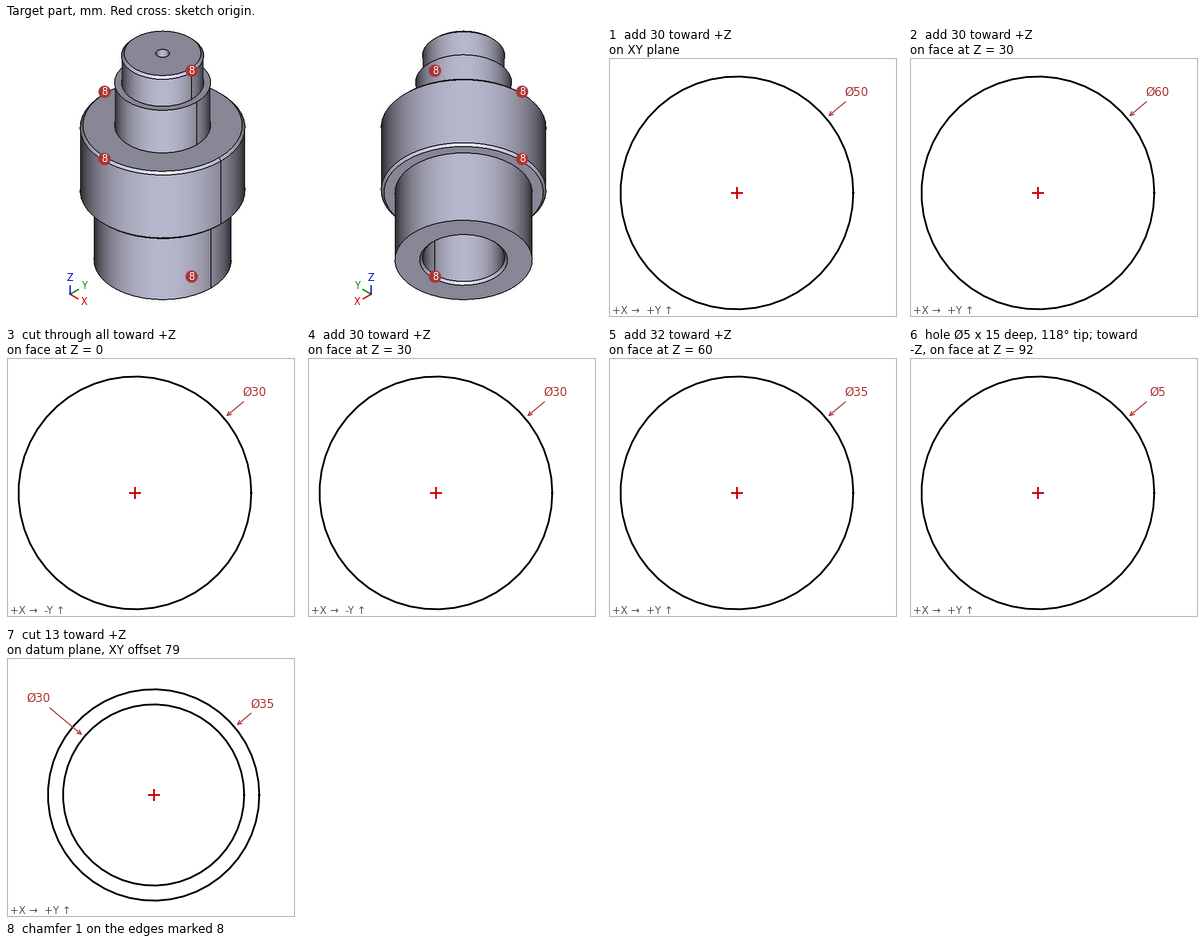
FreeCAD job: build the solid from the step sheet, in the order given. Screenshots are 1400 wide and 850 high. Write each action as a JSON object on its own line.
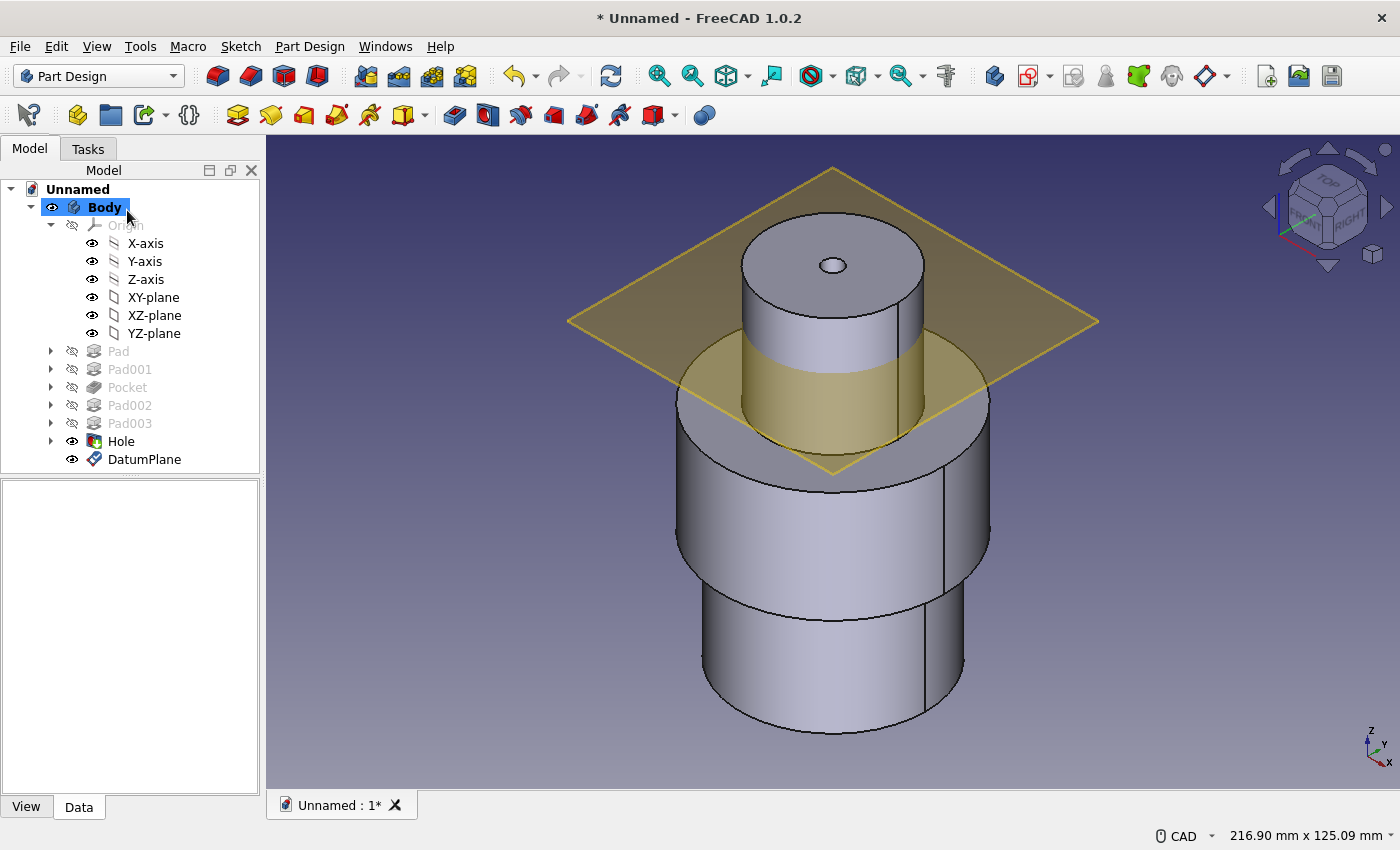
{"action": "left_click", "coordinate": [117, 459]}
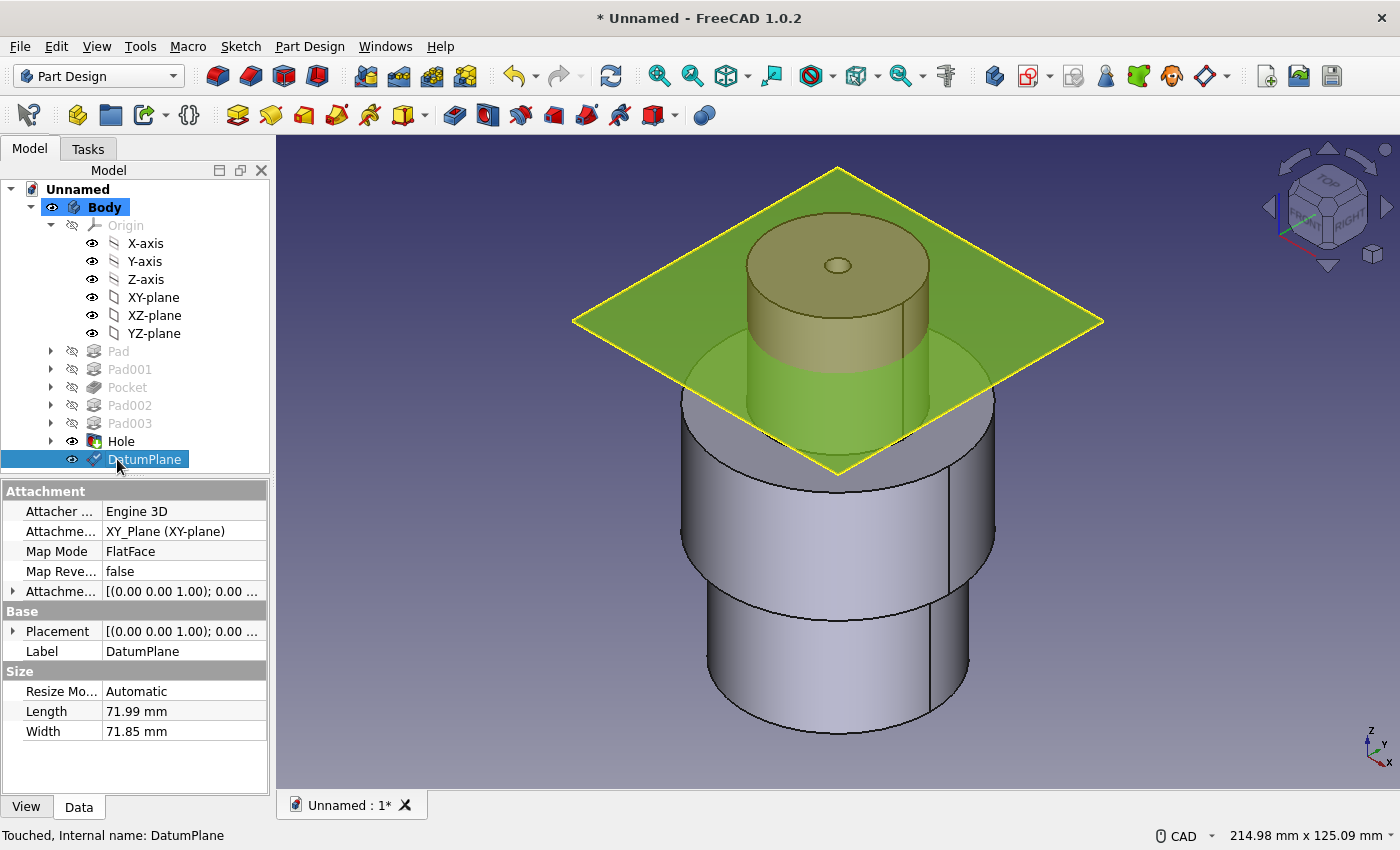
{"action": "left_click", "coordinate": [1028, 76]}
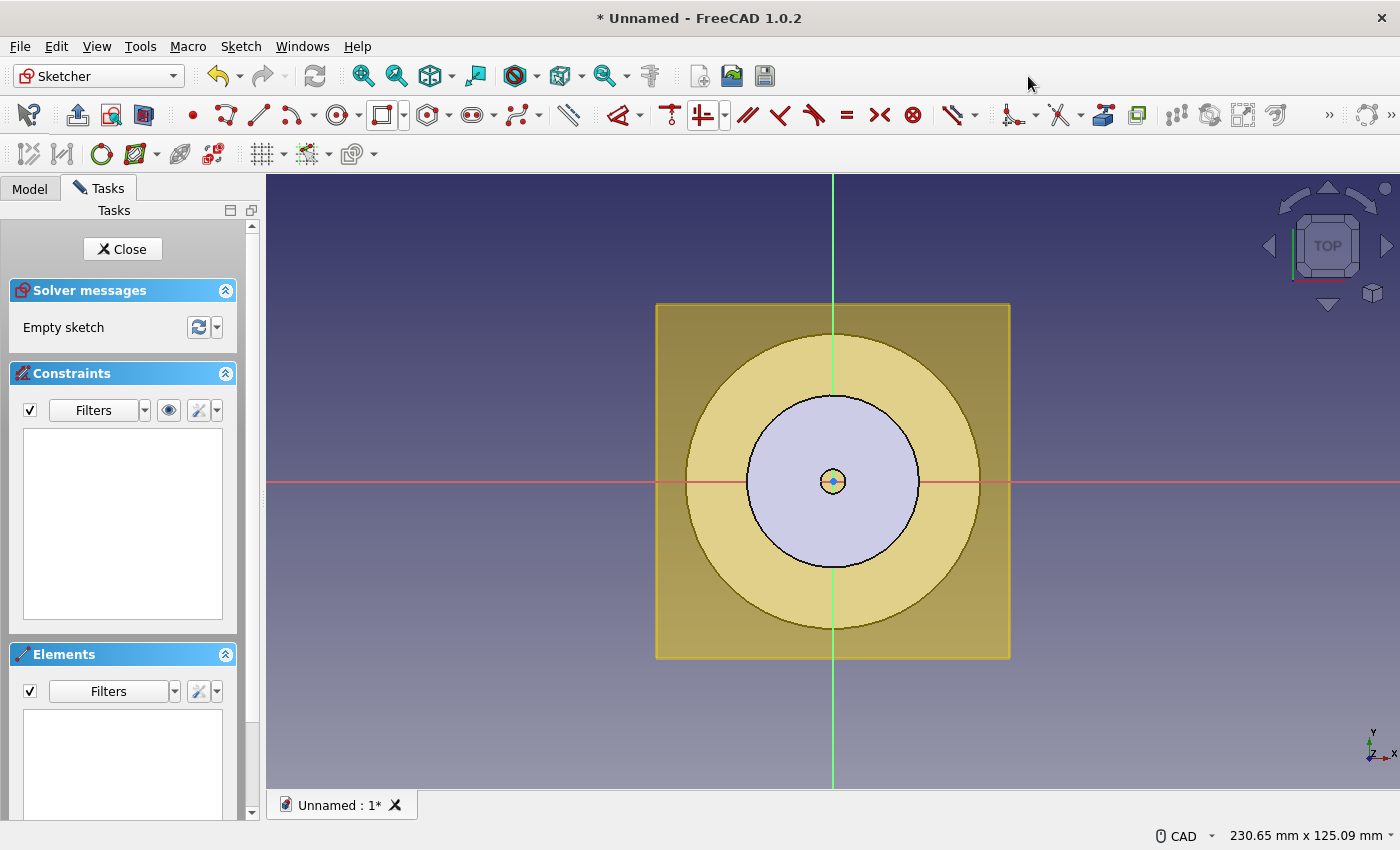
{"action": "left_click", "coordinate": [144, 116]}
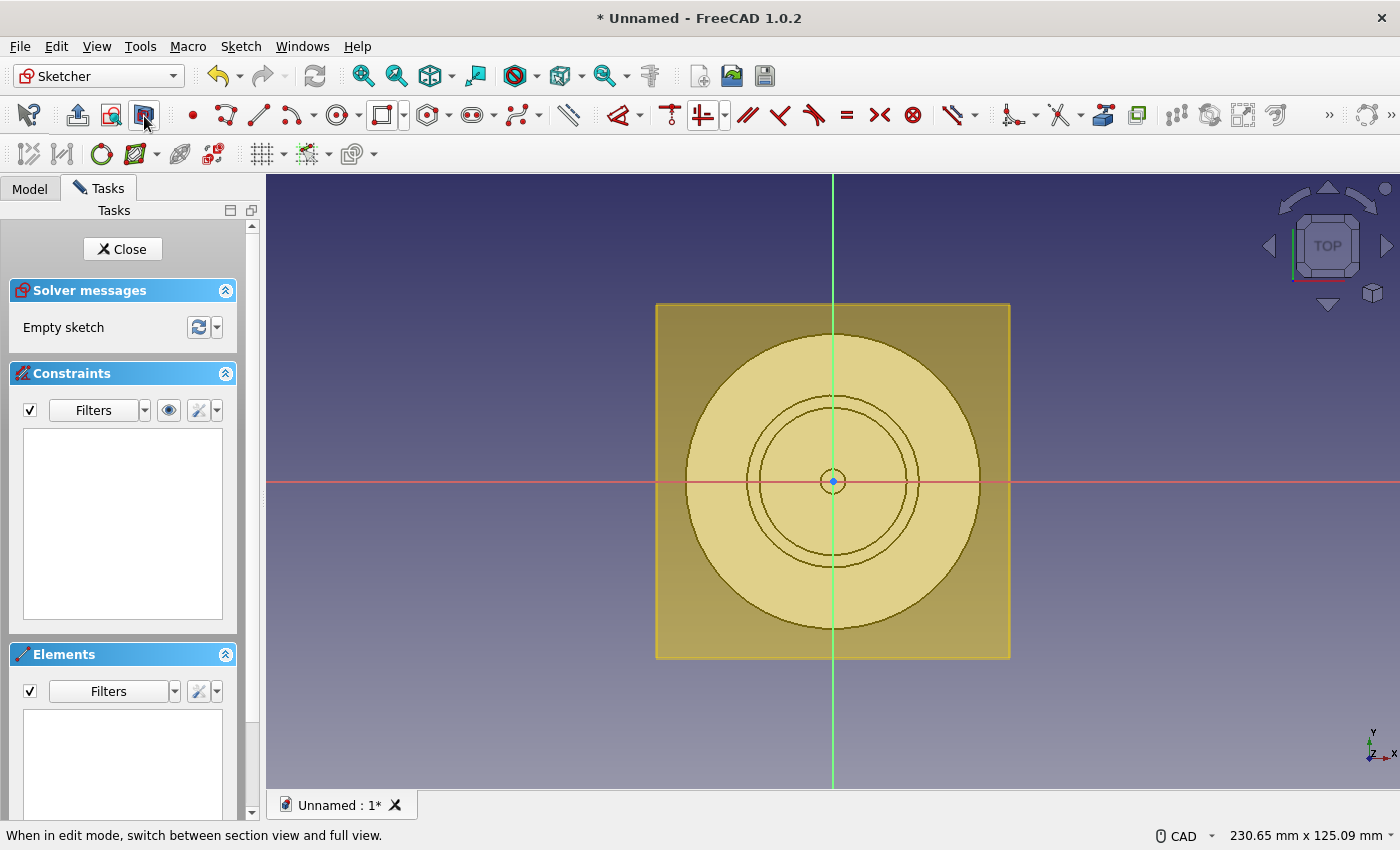
{"action": "scroll", "coordinate": [889, 482], "scroll_direction": "up", "scroll_amount": 4}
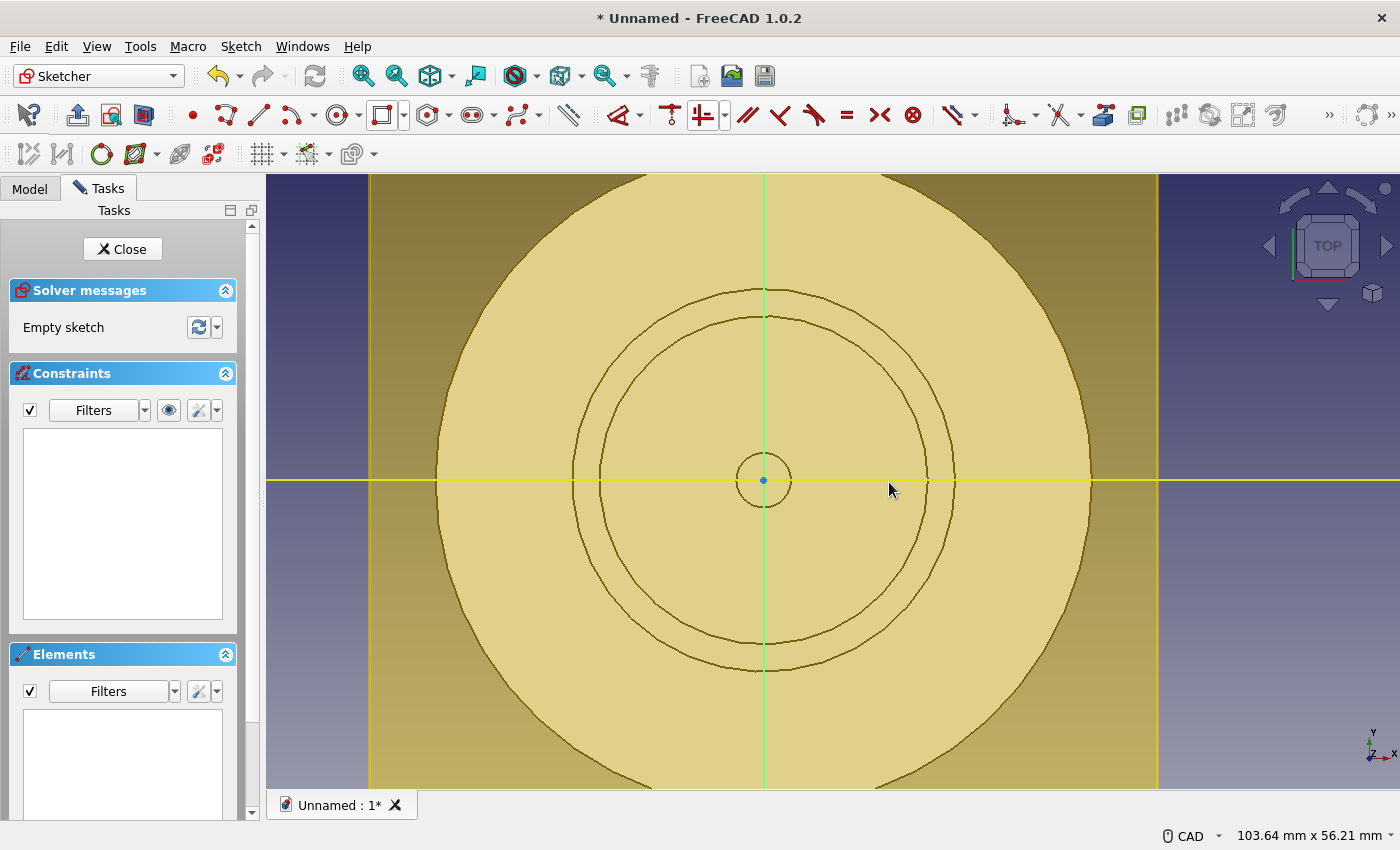
{"action": "key", "text": "g c"}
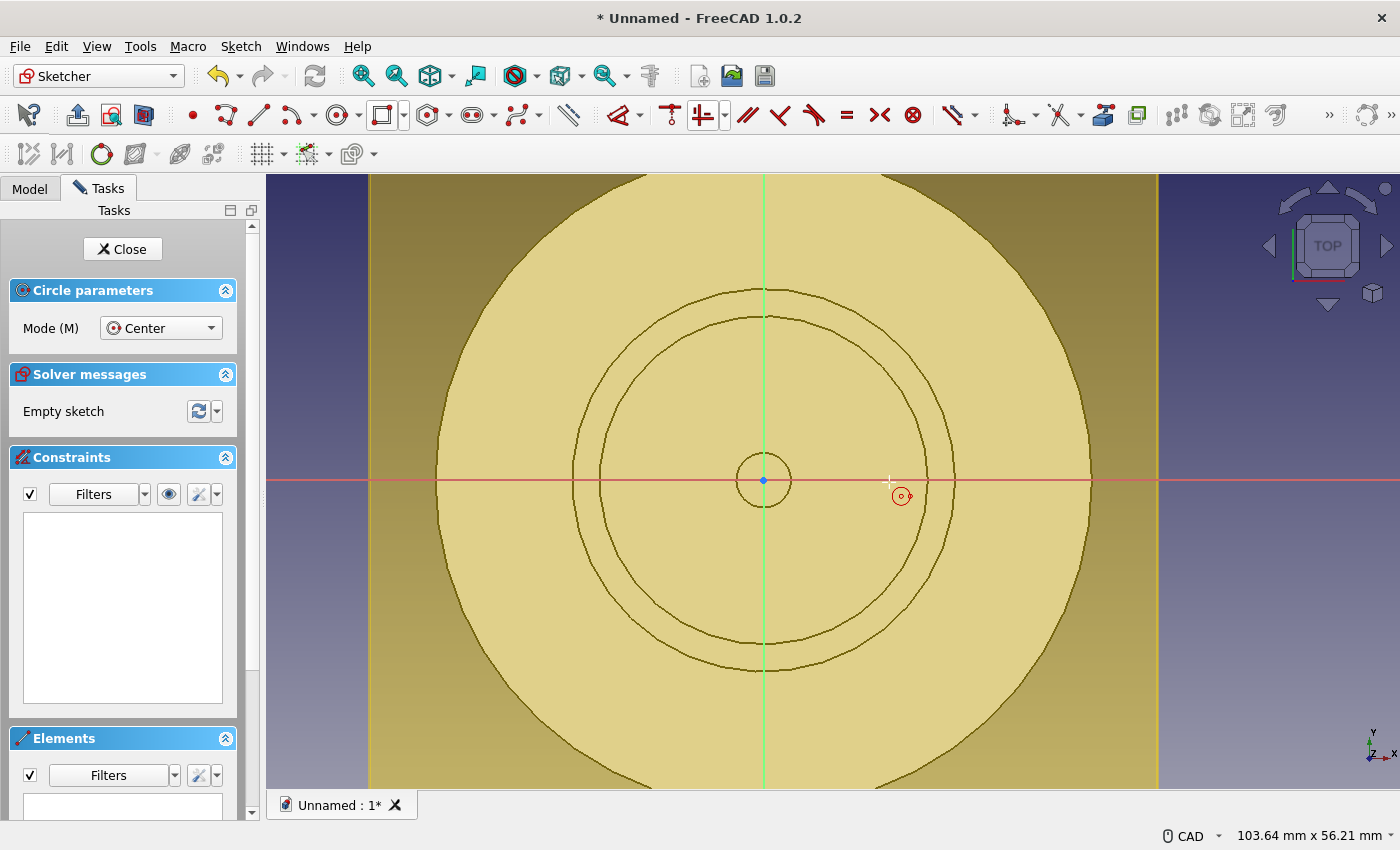
{"action": "left_click", "coordinate": [764, 480]}
{"action": "left_click", "coordinate": [899, 345]}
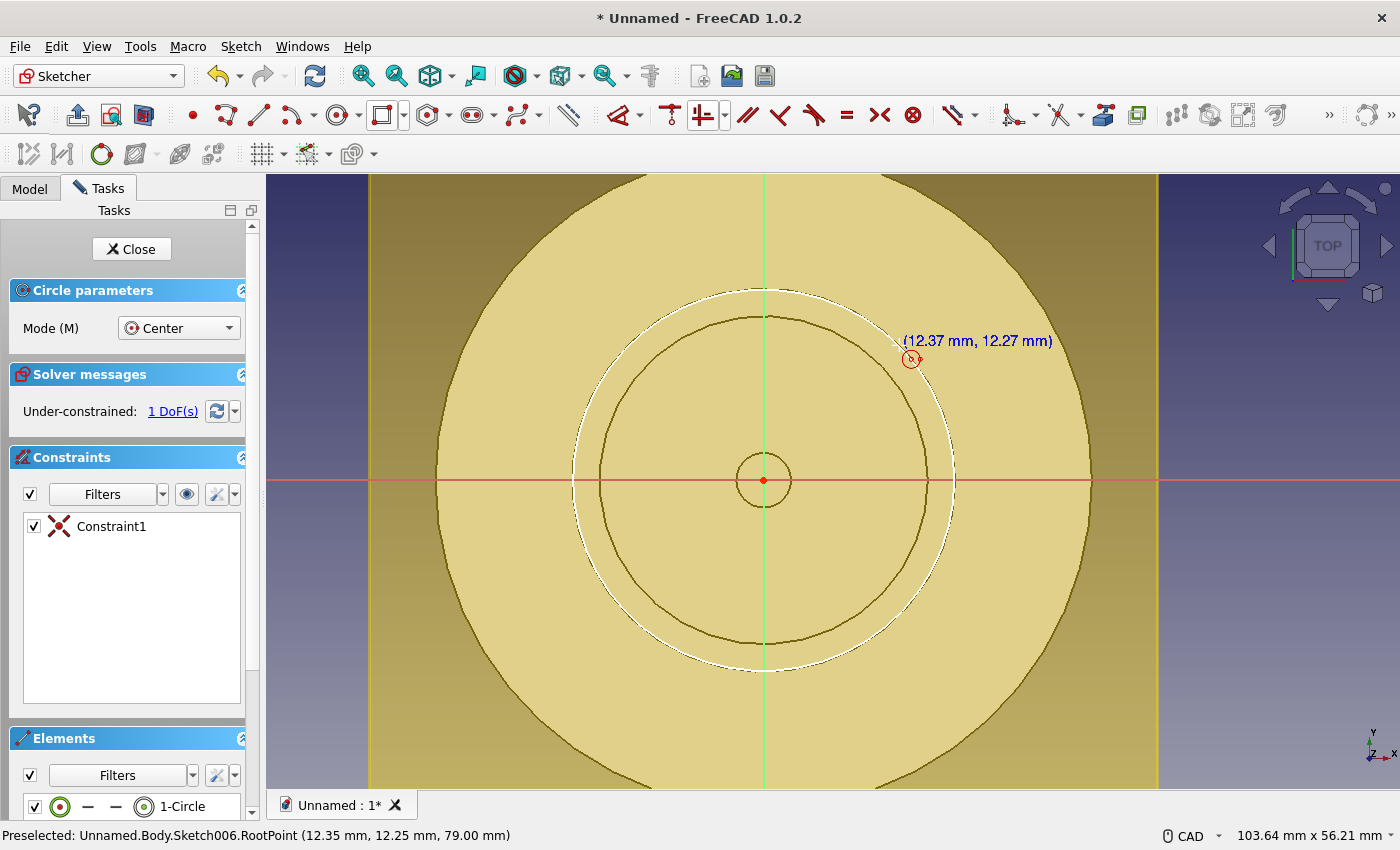
{"action": "left_click", "coordinate": [764, 480]}
{"action": "left_click", "coordinate": [880, 364]}
{"action": "key", "text": "Escape"}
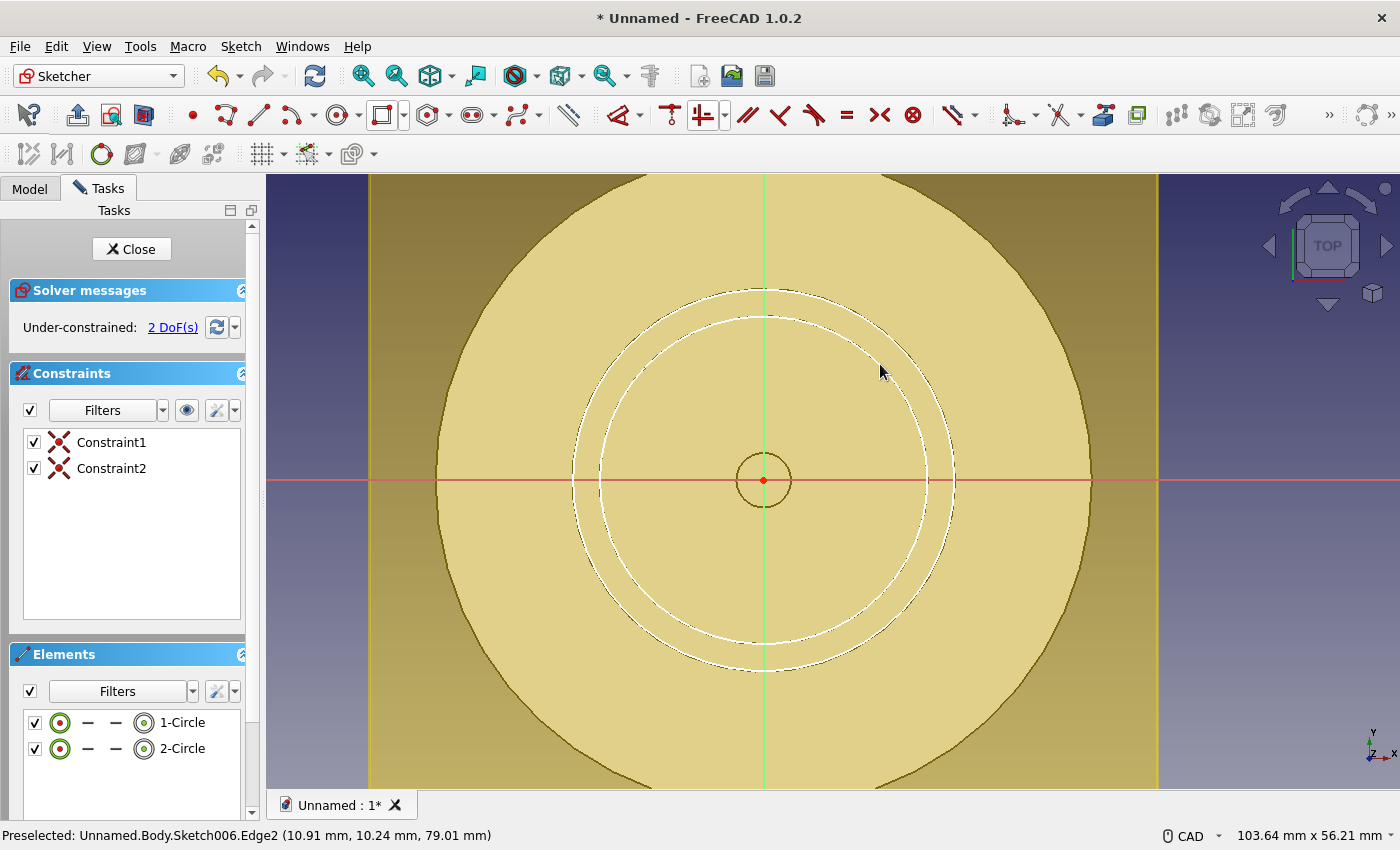
{"action": "key", "text": "d"}